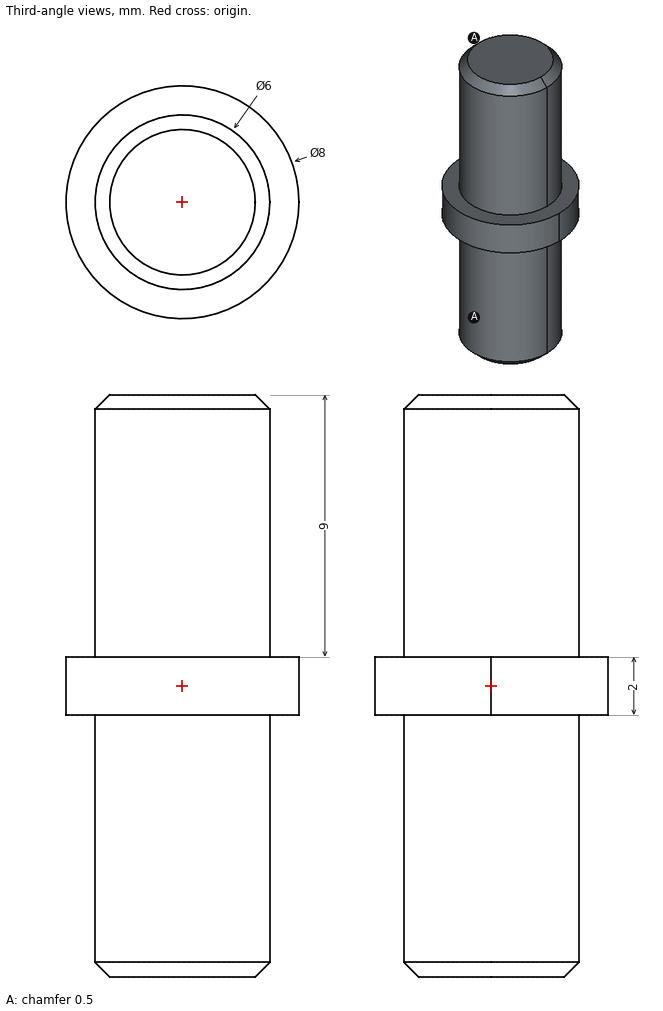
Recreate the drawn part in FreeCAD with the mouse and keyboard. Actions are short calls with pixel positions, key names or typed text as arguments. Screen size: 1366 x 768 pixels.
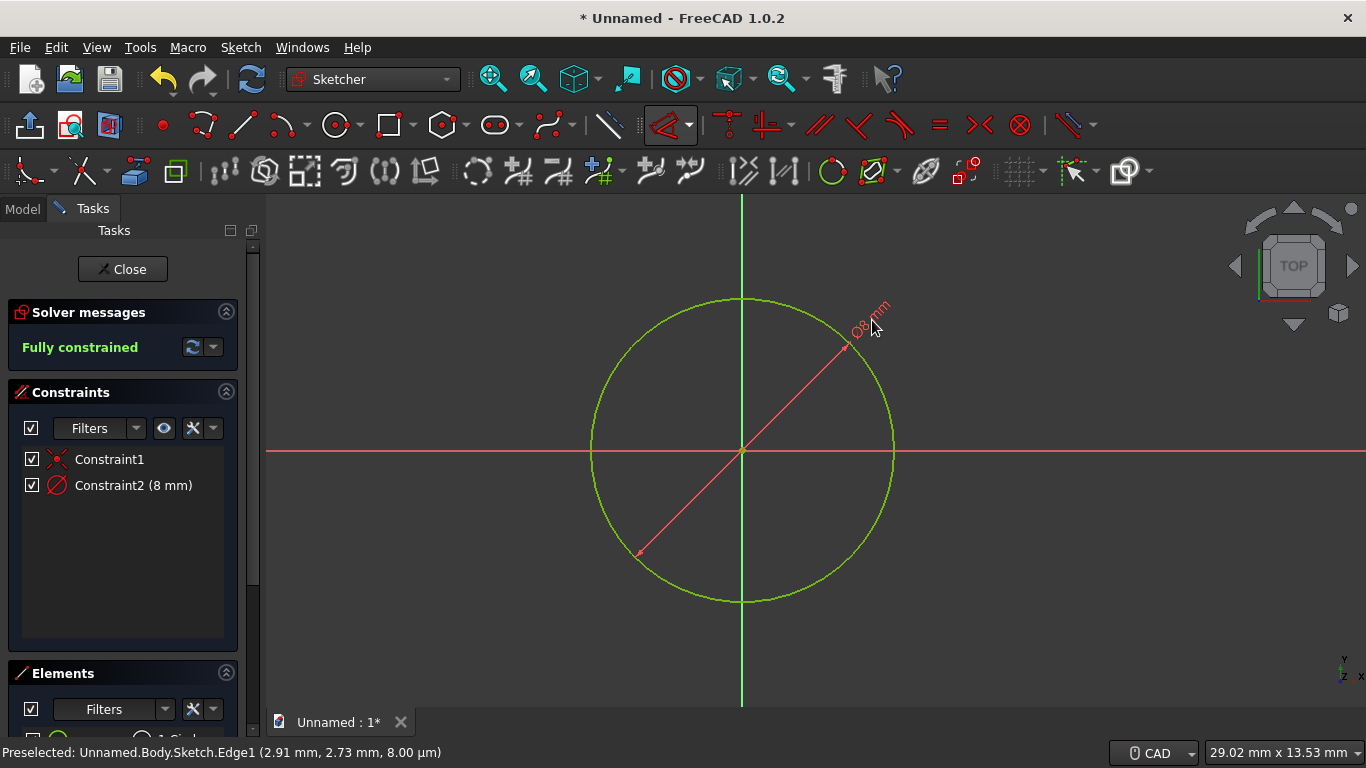
click(123, 269)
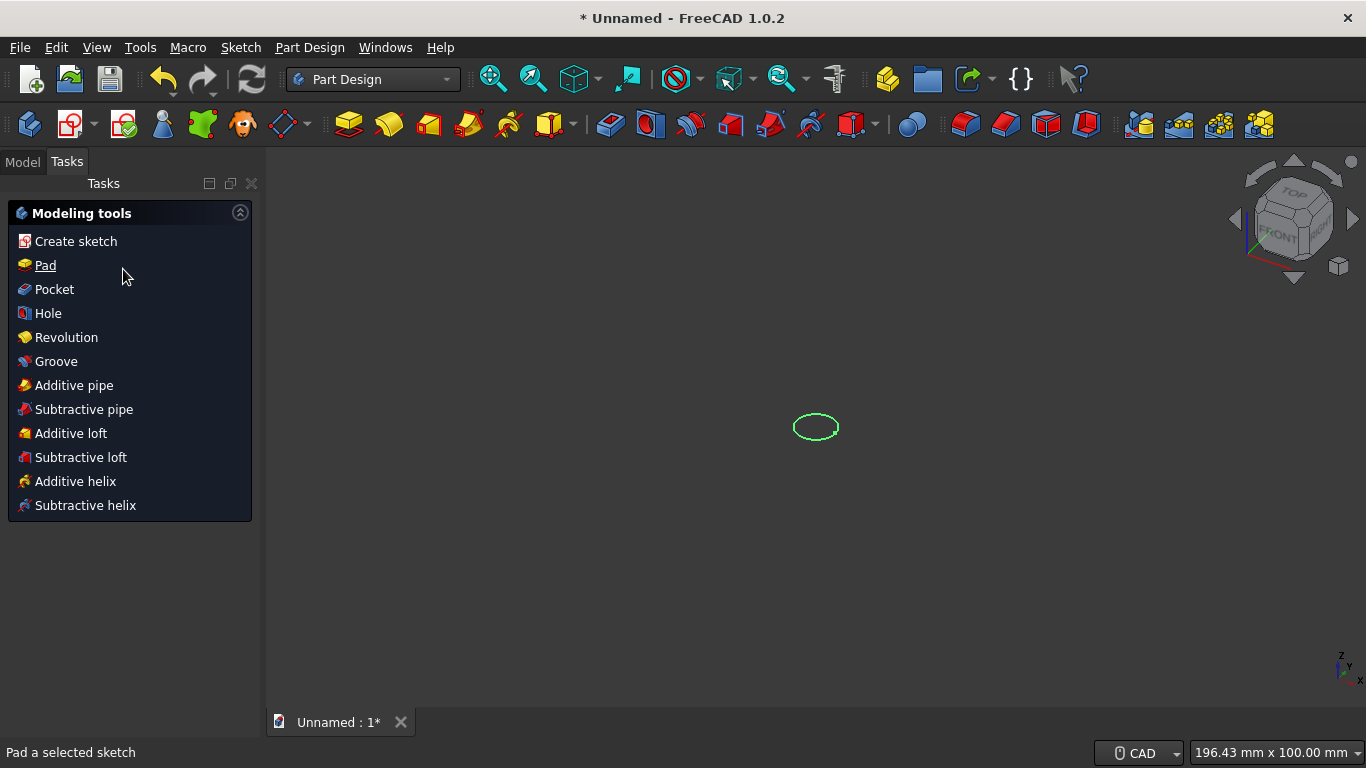
click(350, 124)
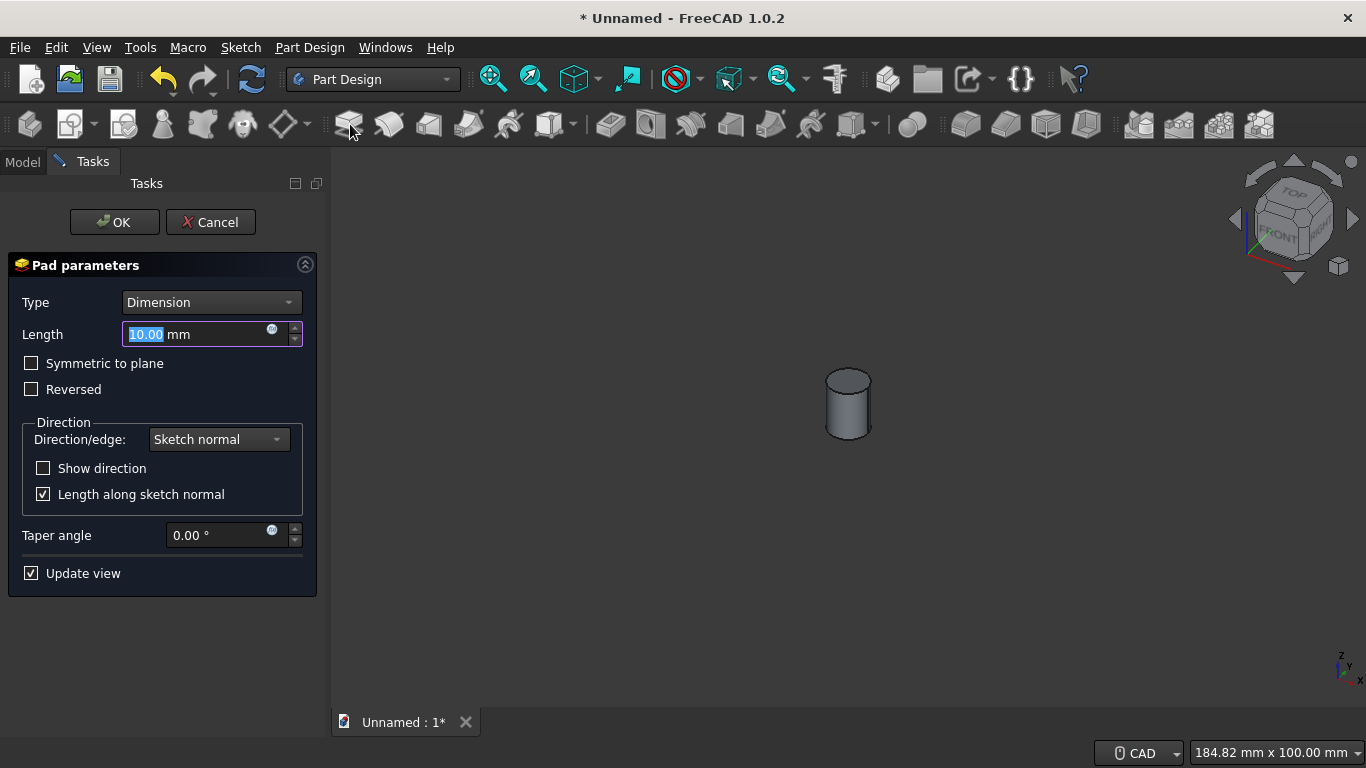
text(2)
key(Tab)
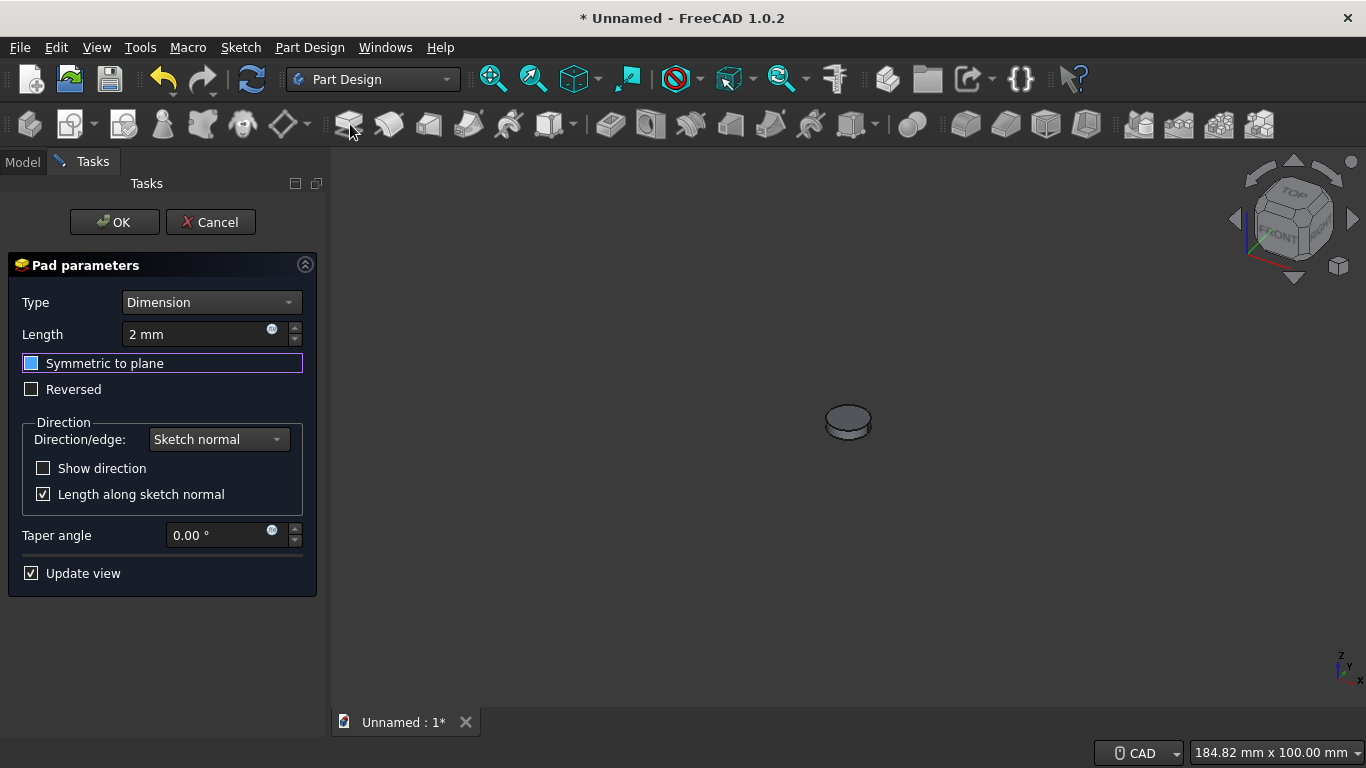
click(30, 363)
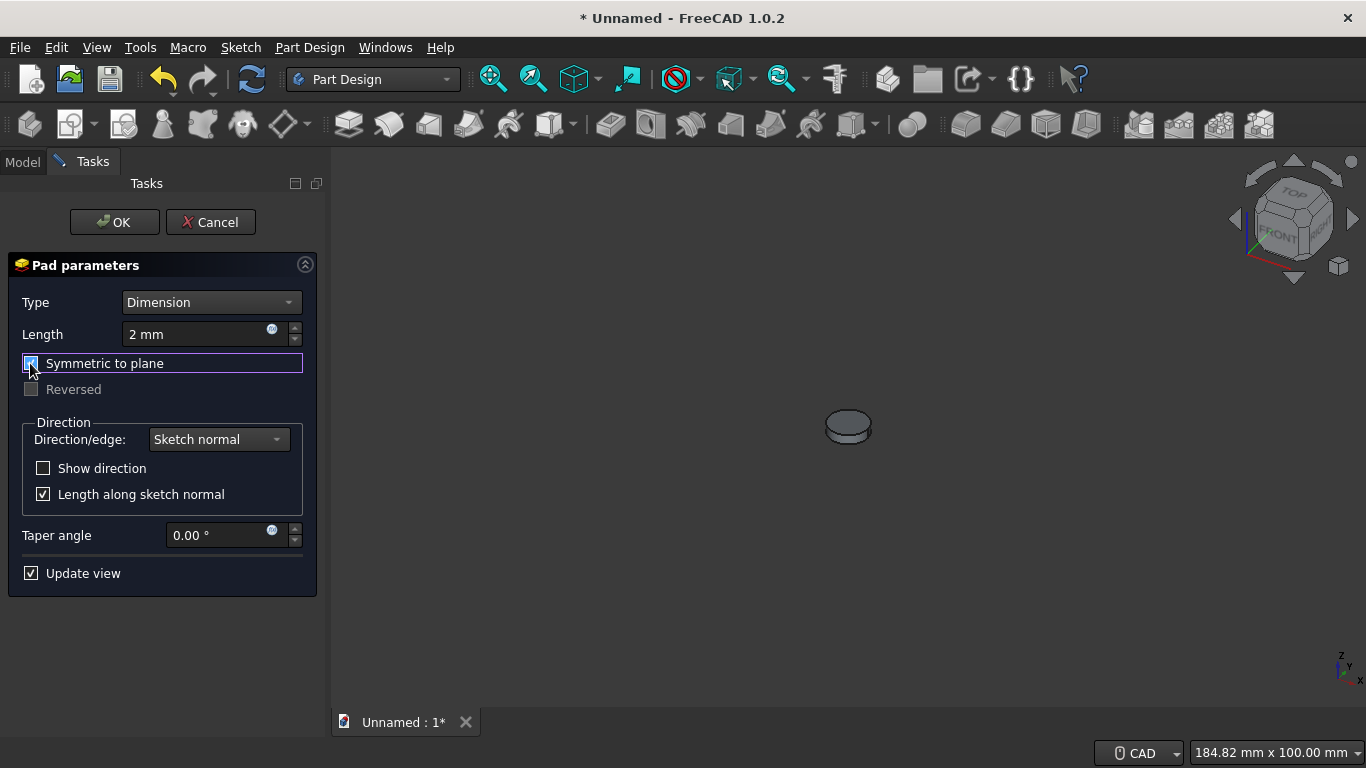
click(115, 222)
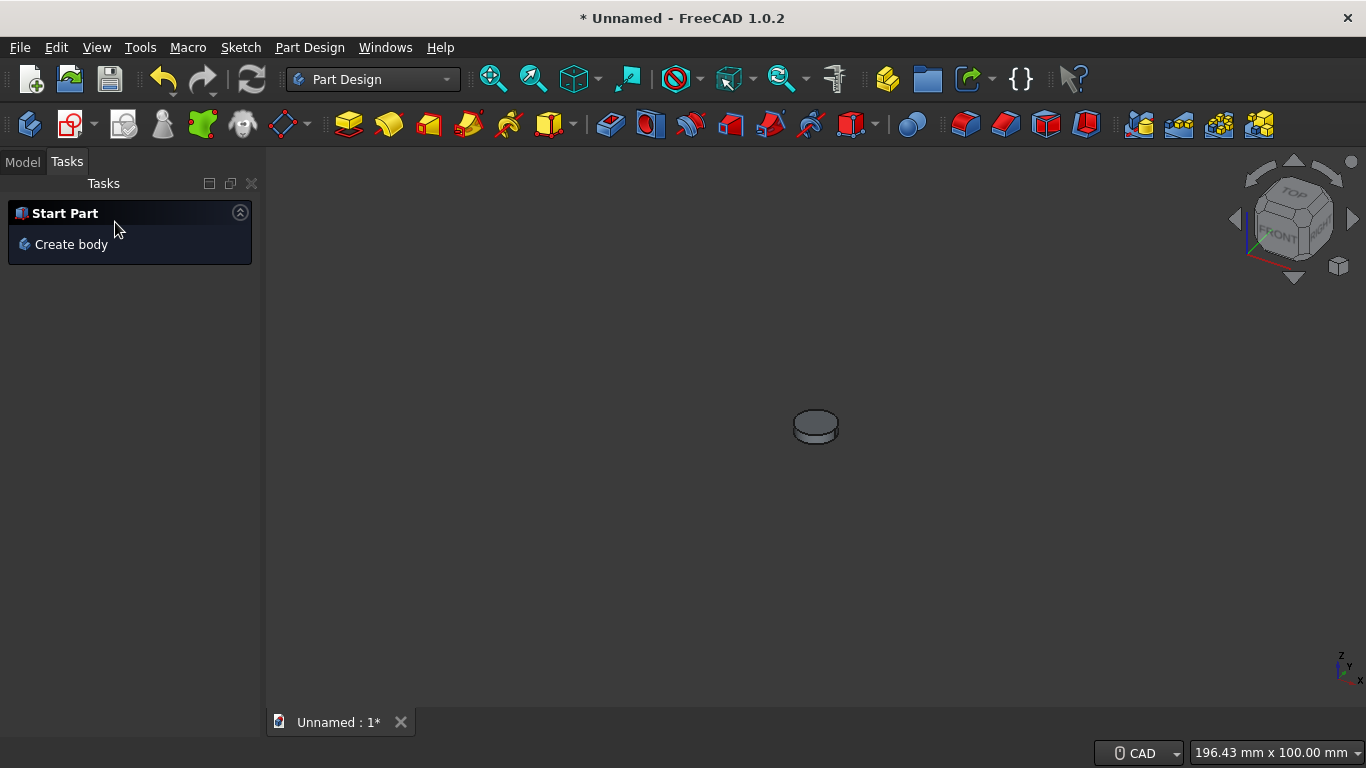
click(494, 80)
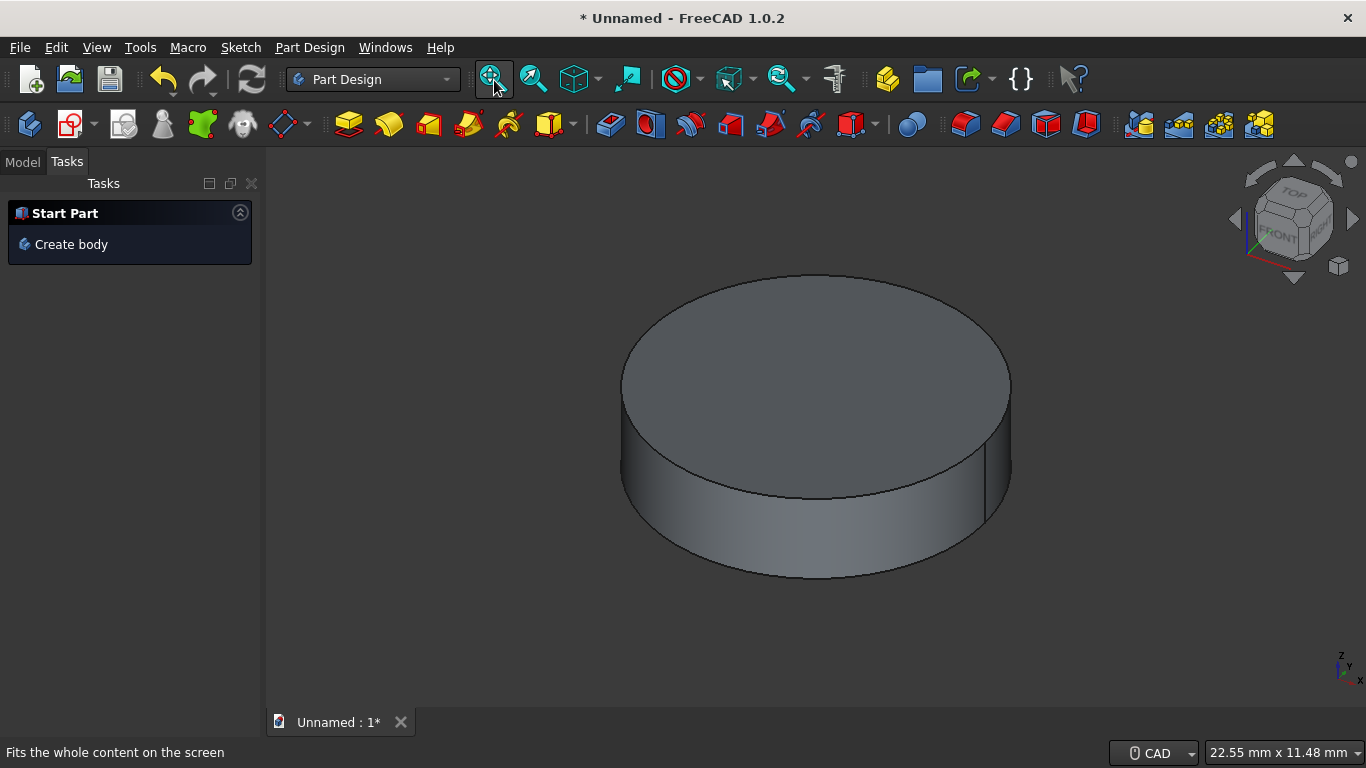
click(816, 386)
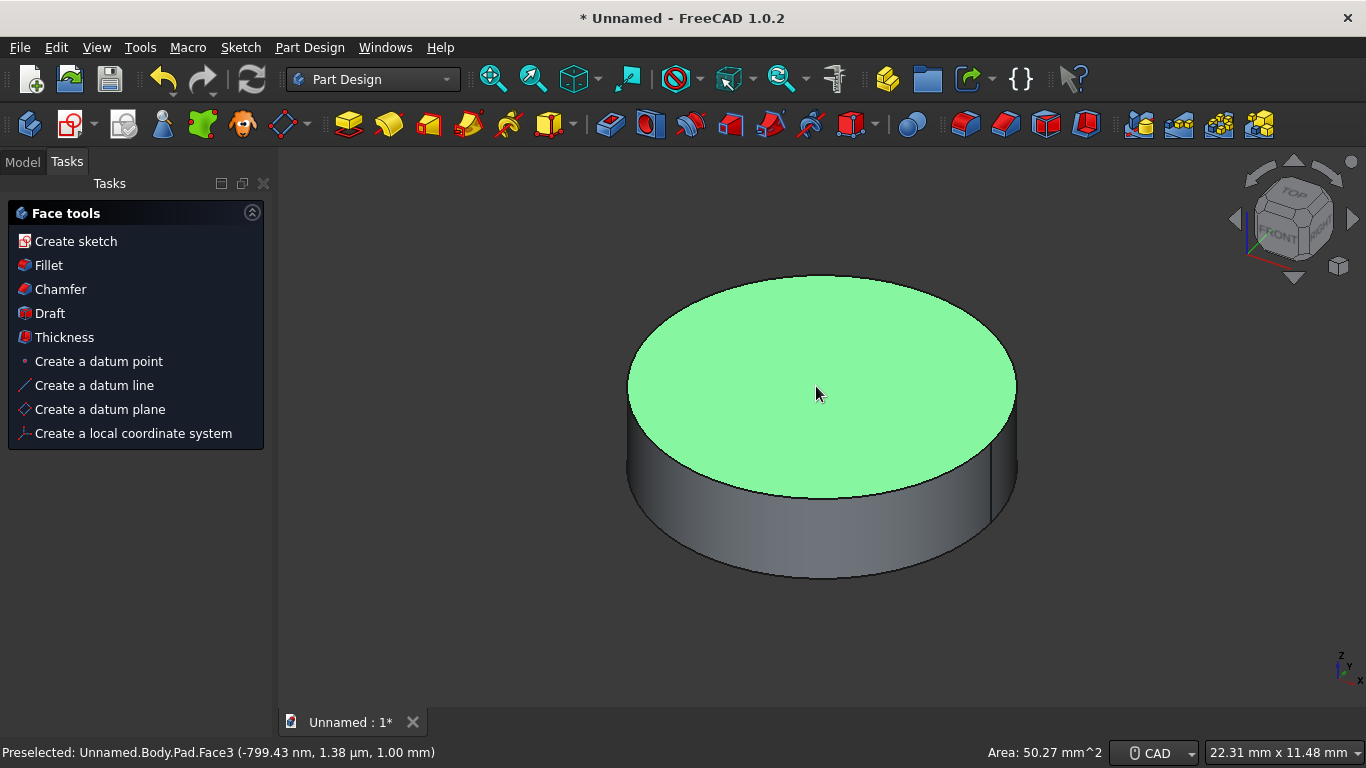
click(70, 124)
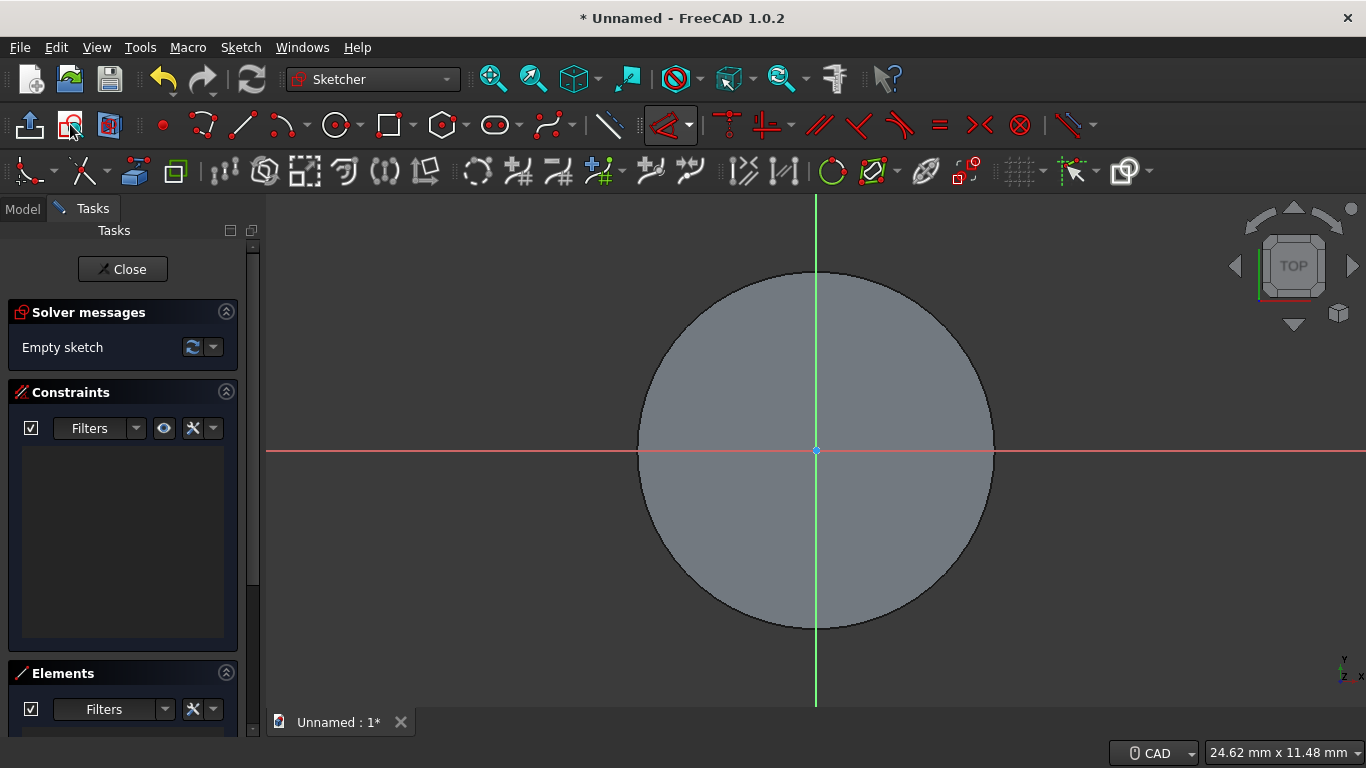
key(g)
key(c)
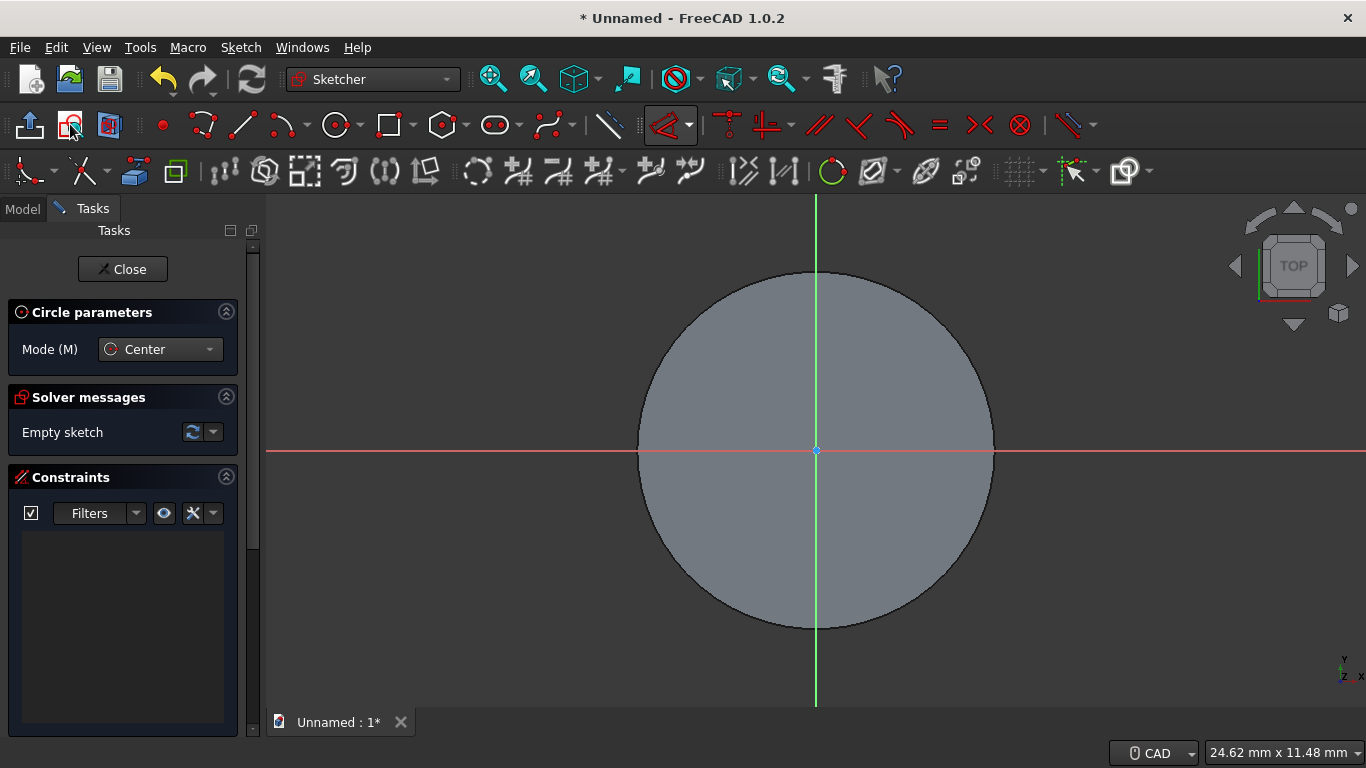
click(816, 450)
click(911, 356)
key(Escape)